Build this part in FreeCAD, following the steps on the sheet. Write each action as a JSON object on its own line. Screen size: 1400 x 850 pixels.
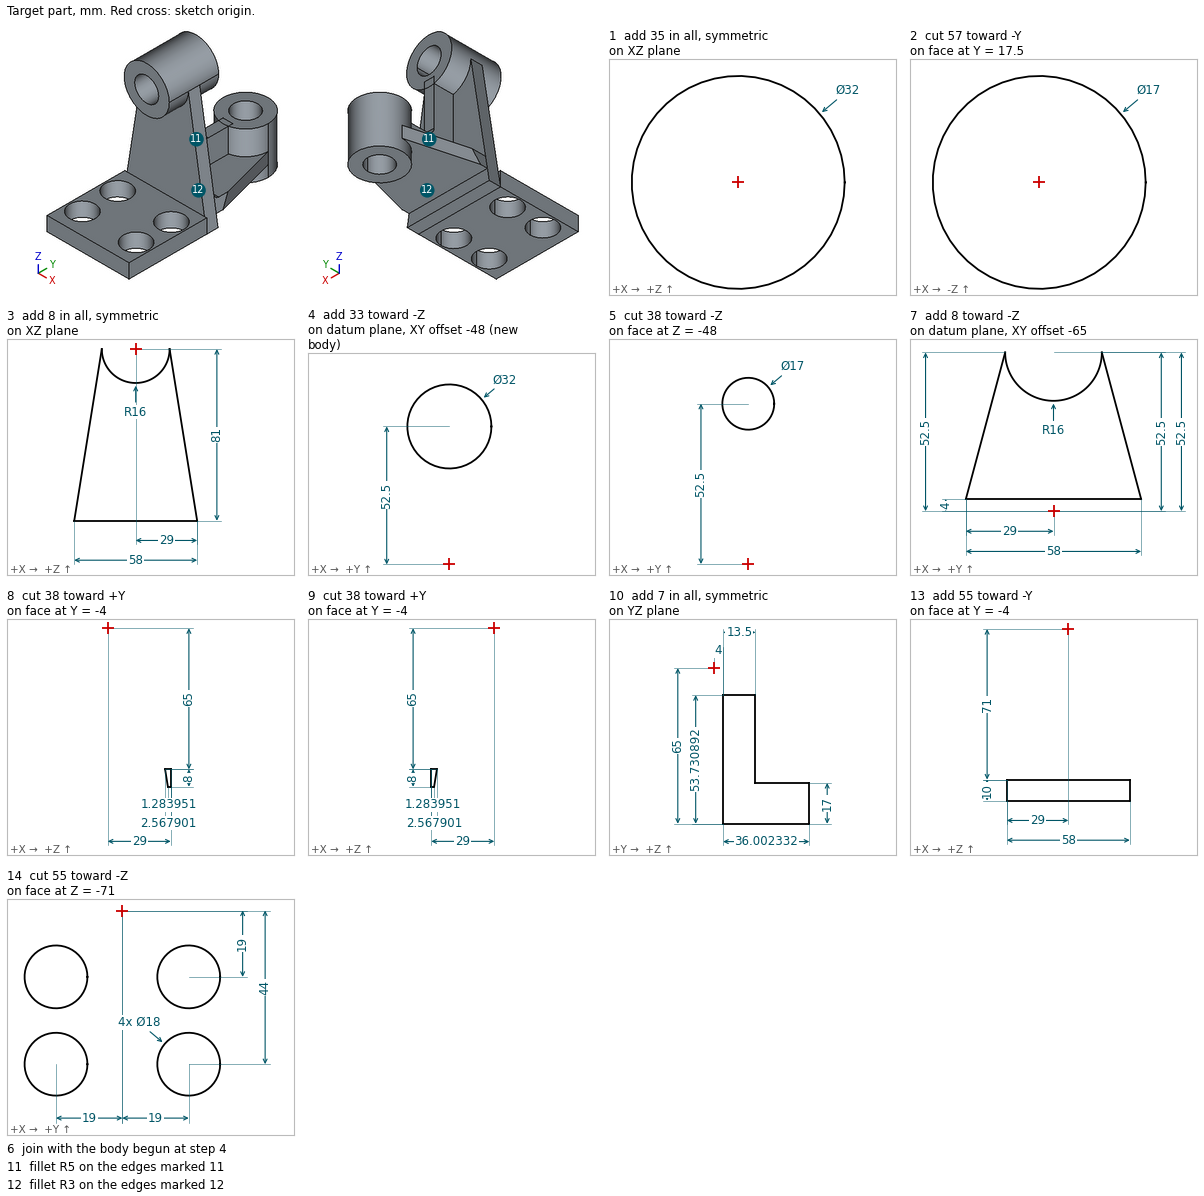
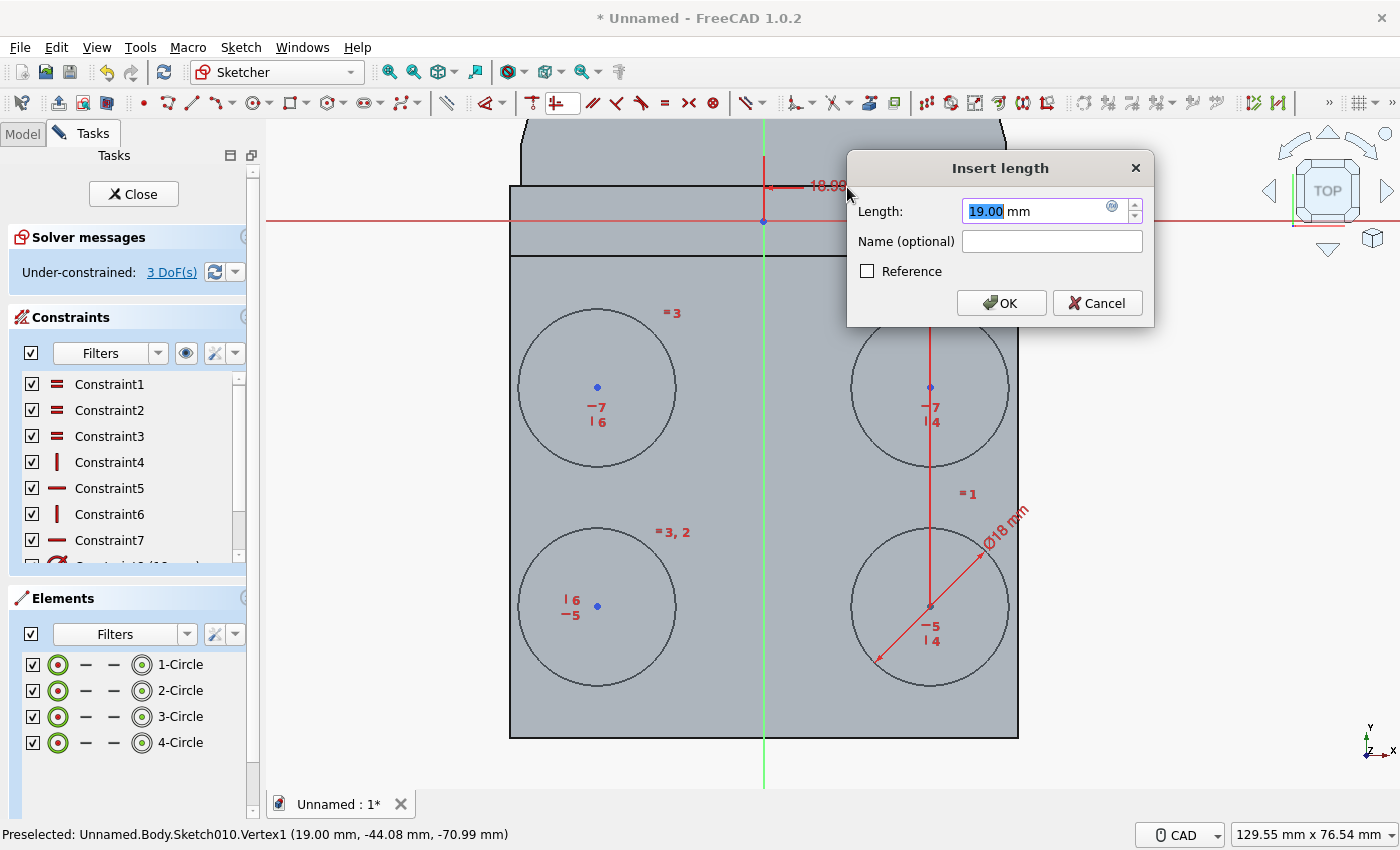
{"action": "type", "text": "19"}
{"action": "key", "text": "Return"}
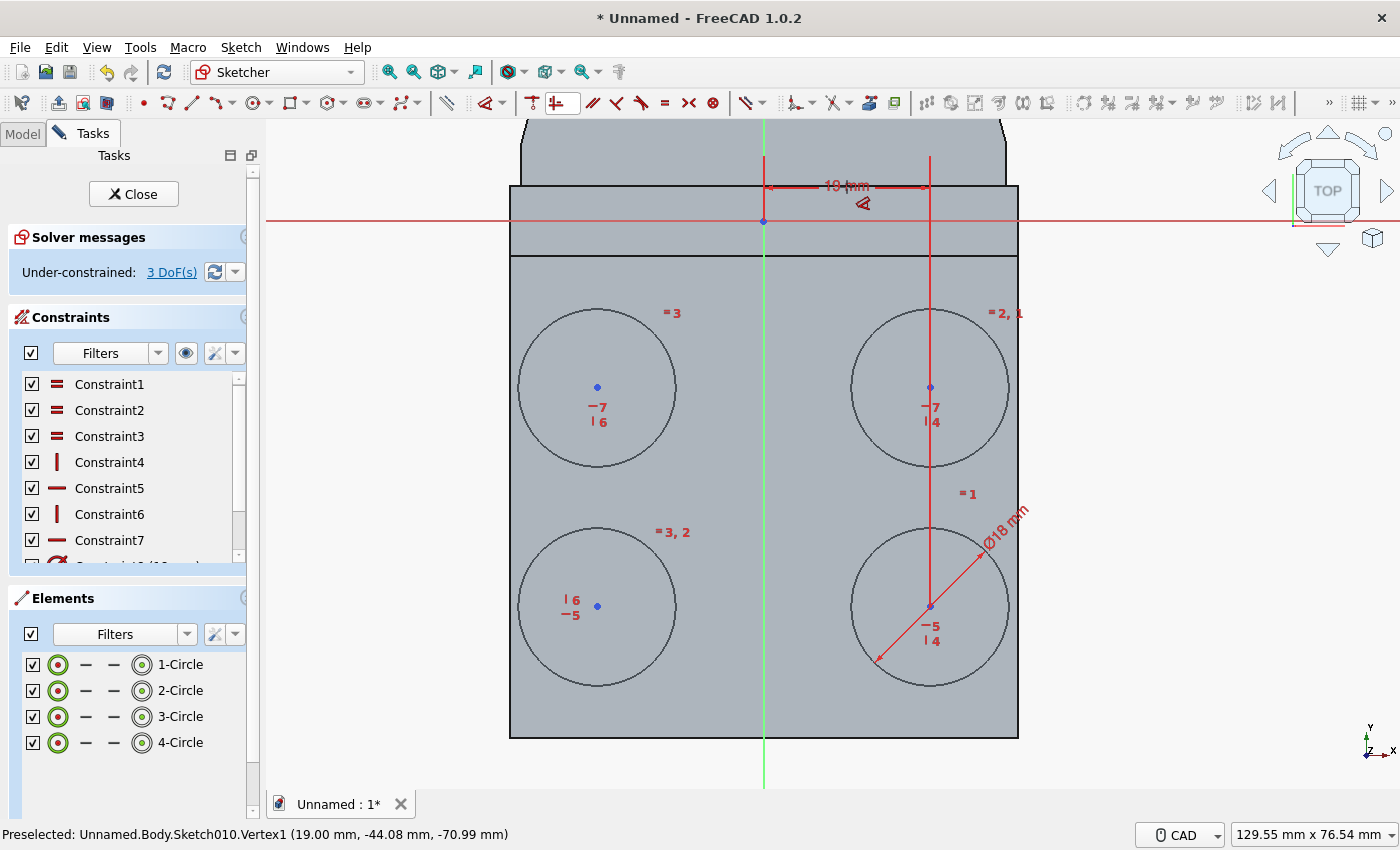
{"action": "left_click", "coordinate": [930, 607]}
{"action": "left_click", "coordinate": [964, 414]}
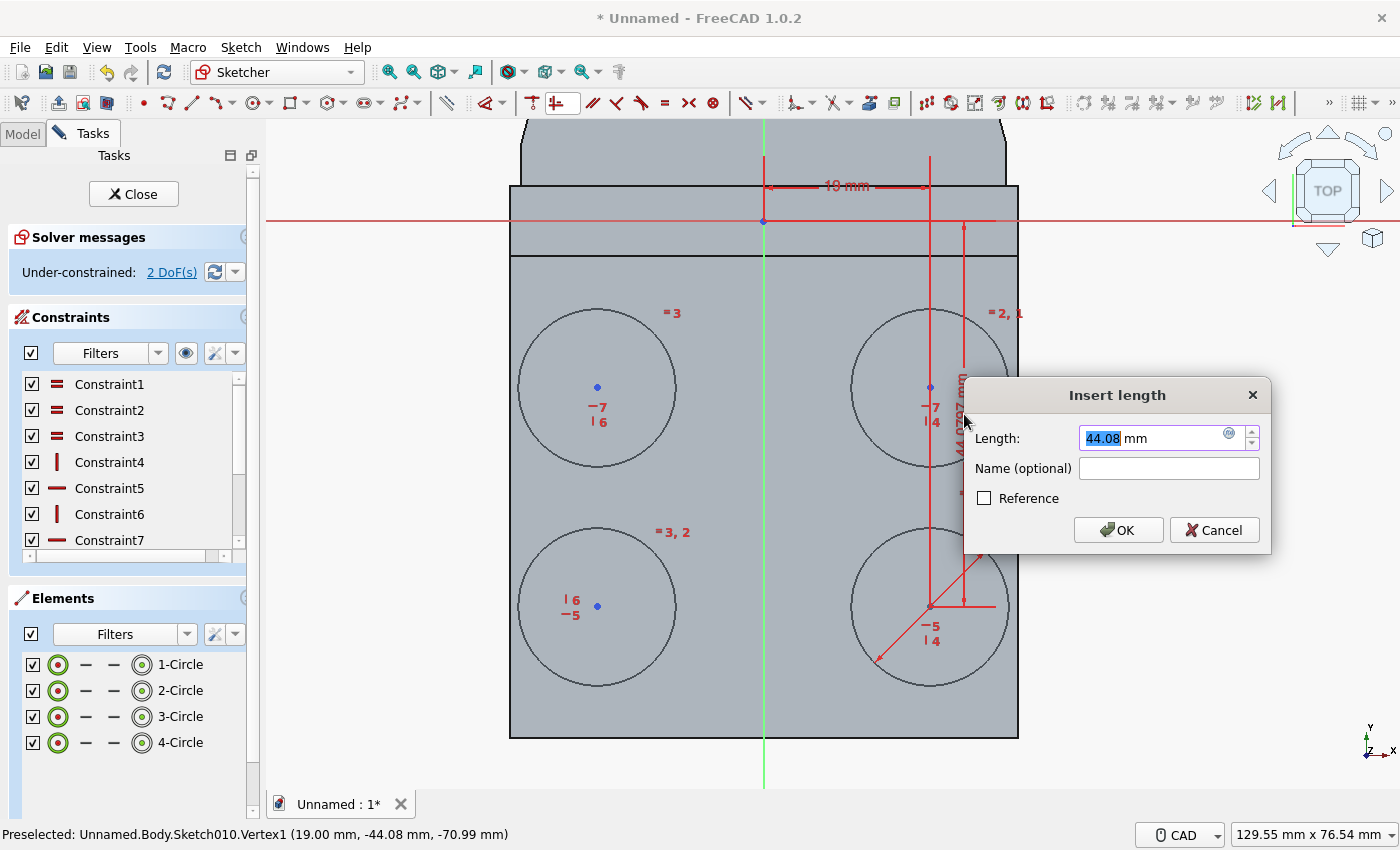
{"action": "type", "text": "44"}
{"action": "key", "text": "Return"}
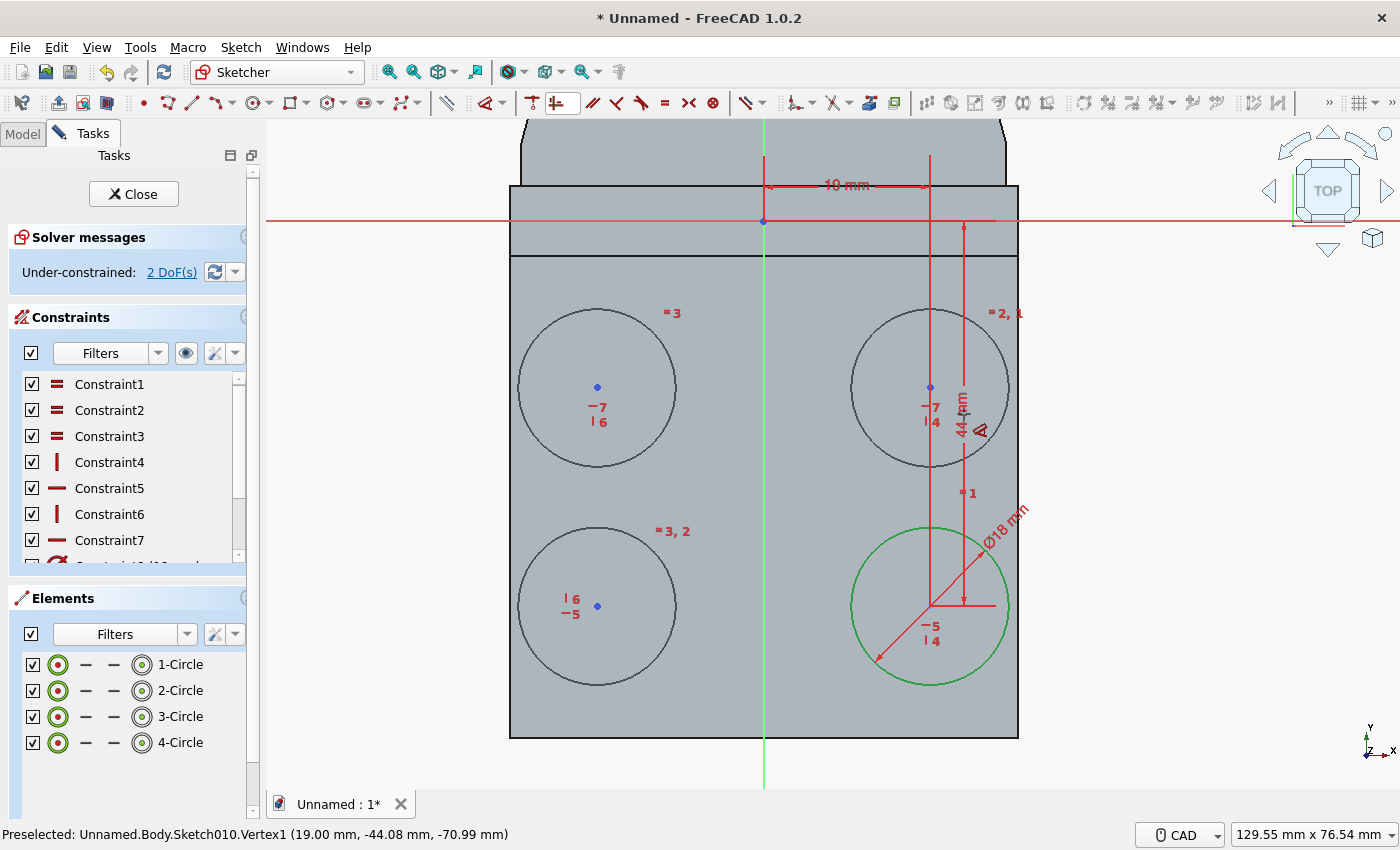
{"action": "left_click", "coordinate": [930, 388]}
{"action": "left_click", "coordinate": [964, 266]}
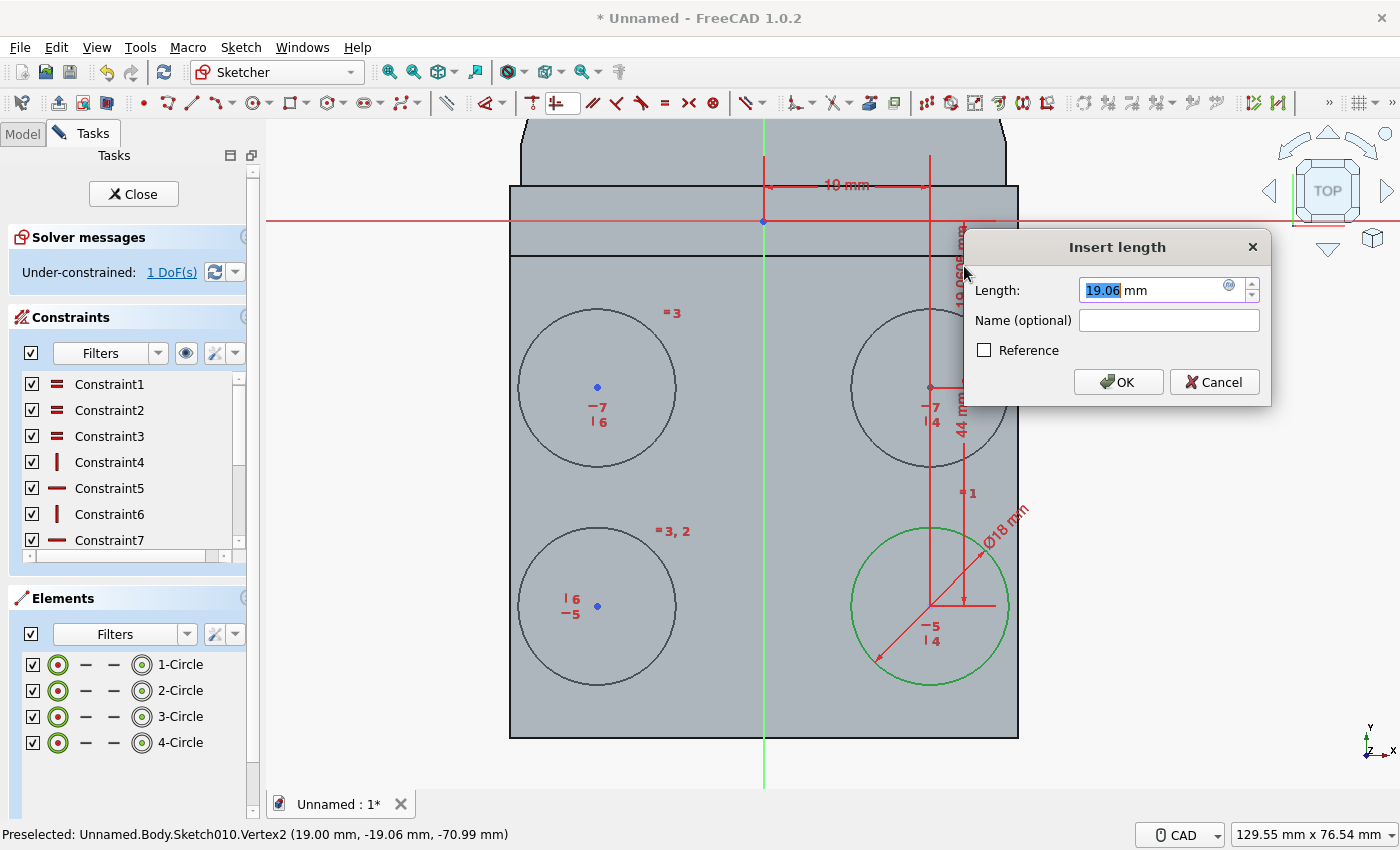
{"action": "type", "text": "19"}
{"action": "key", "text": "Return"}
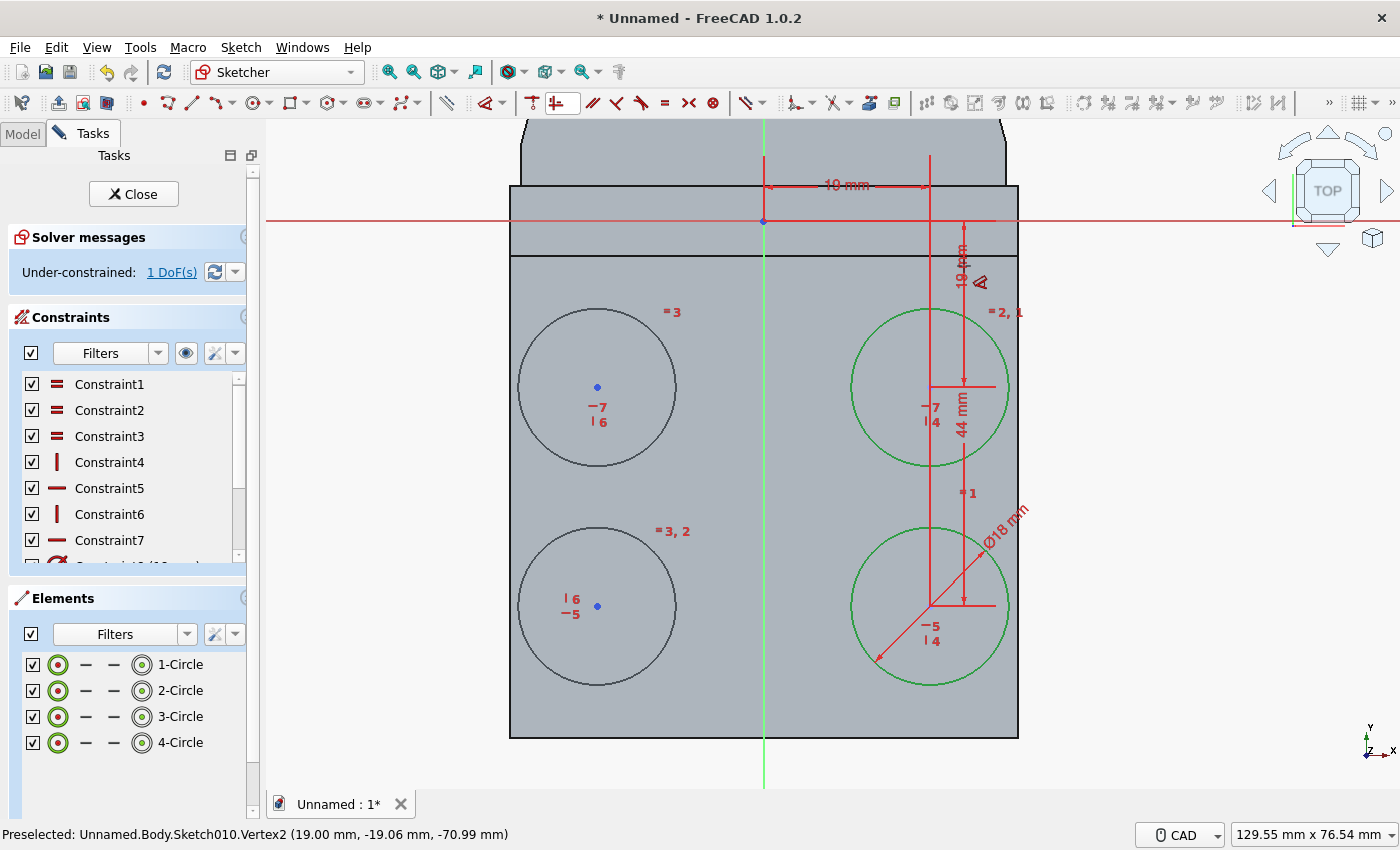
{"action": "left_click", "coordinate": [597, 606]}
{"action": "left_click", "coordinate": [680, 187]}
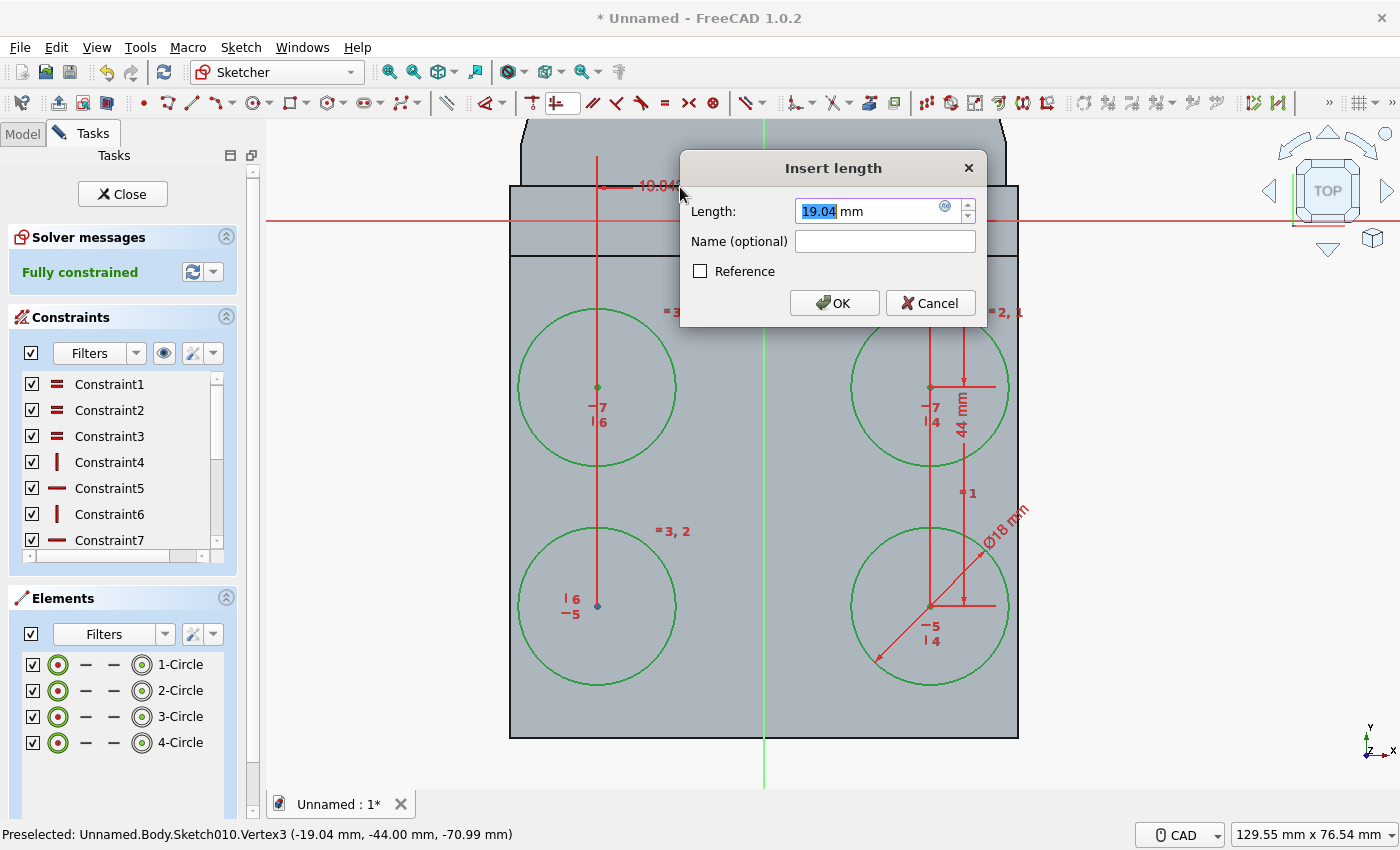
{"action": "type", "text": "19"}
{"action": "key", "text": "Return"}
{"action": "key", "text": "Escape"}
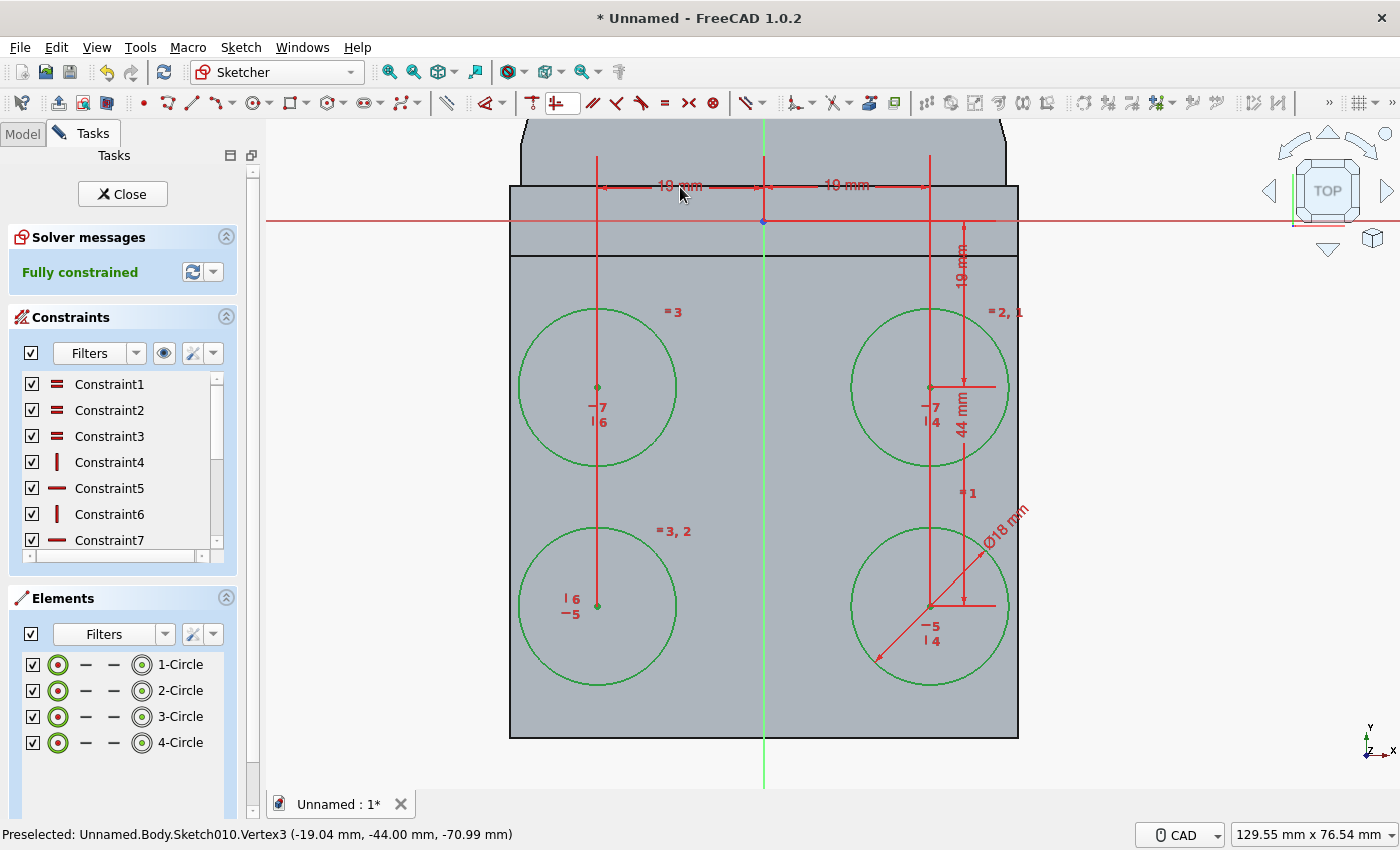
{"action": "left_click", "coordinate": [123, 194]}